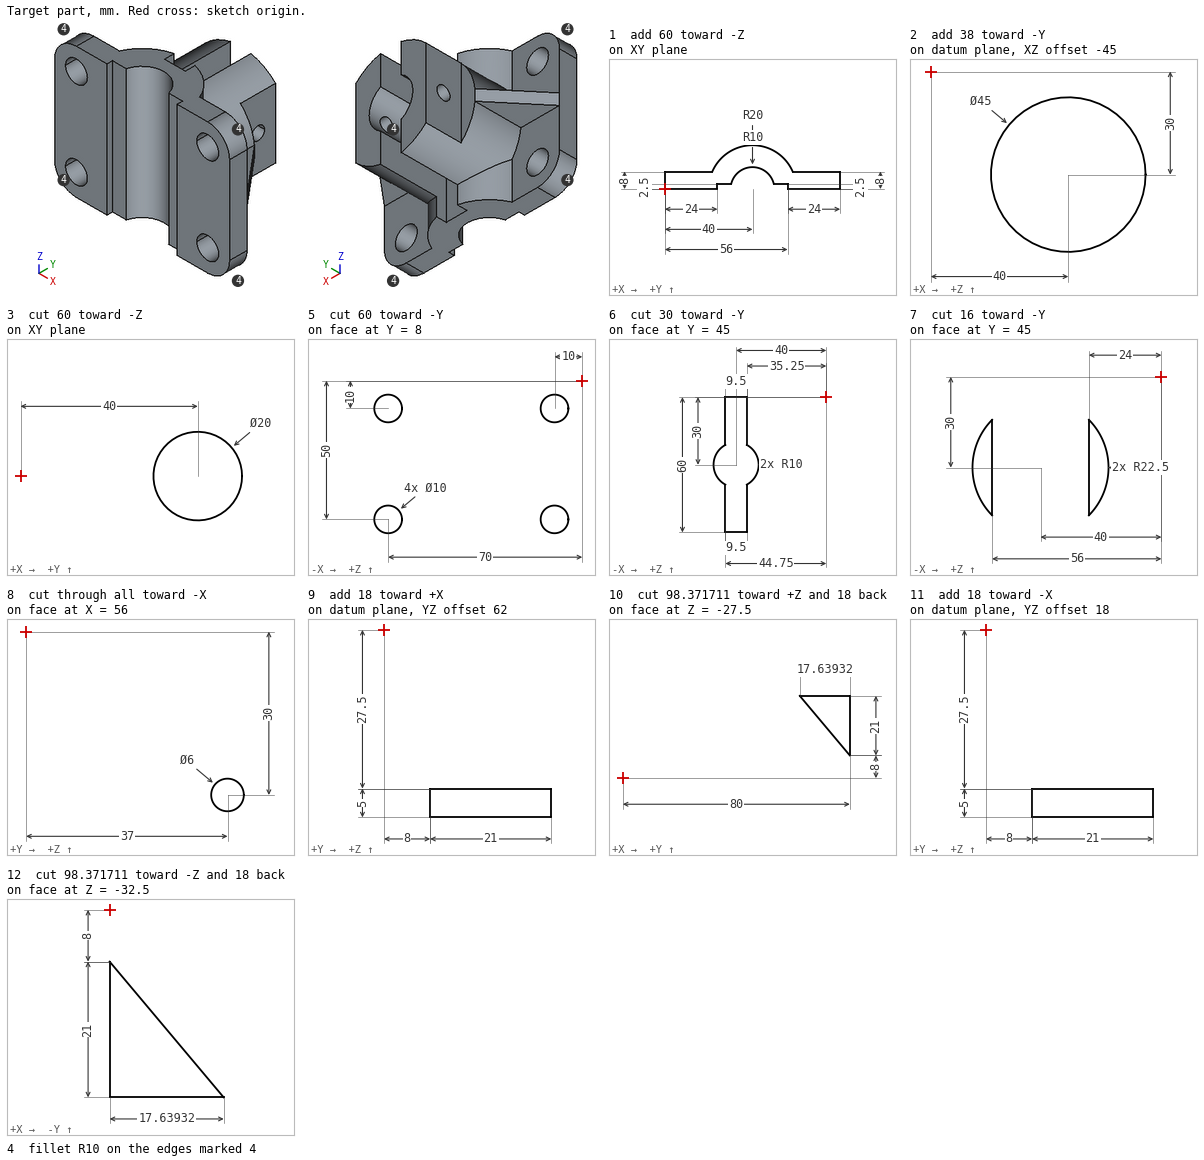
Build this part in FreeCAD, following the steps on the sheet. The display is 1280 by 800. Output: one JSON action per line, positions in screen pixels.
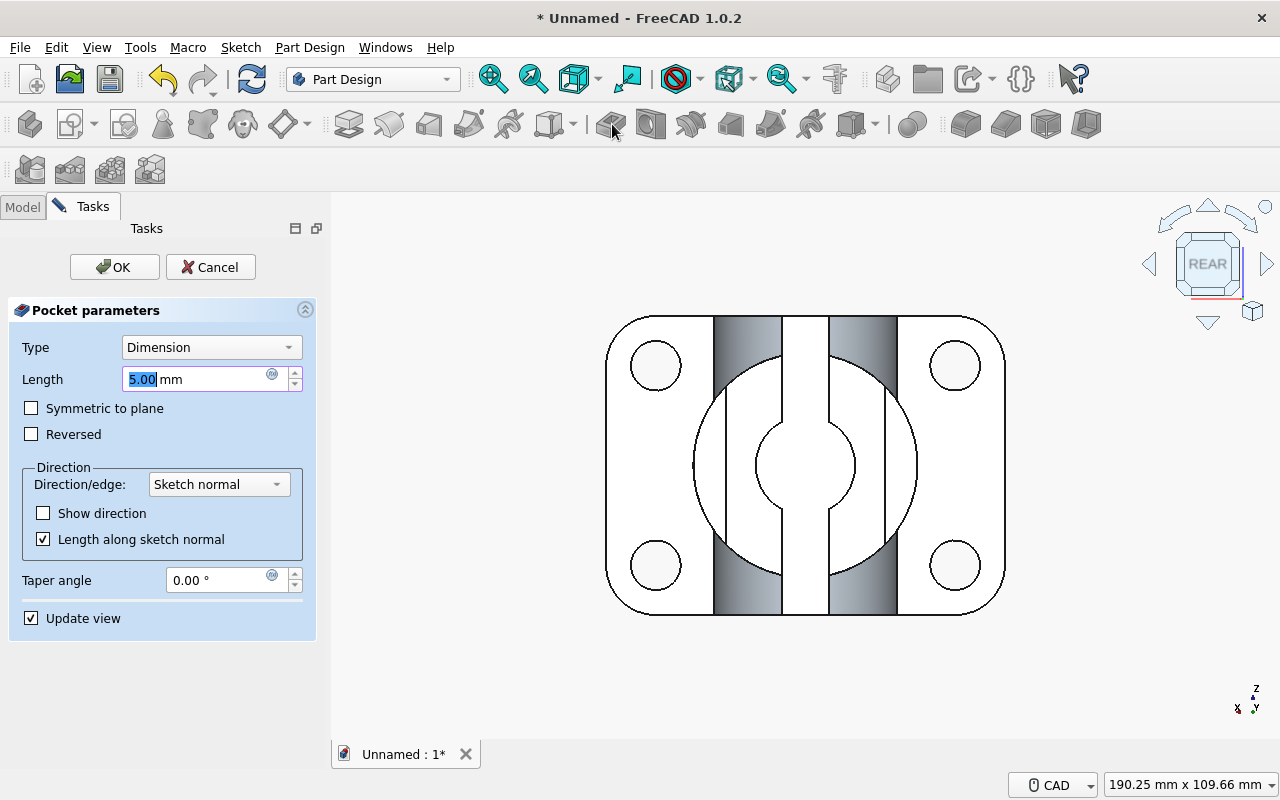
{"action": "type", "text": "16"}
{"action": "key", "text": "Tab"}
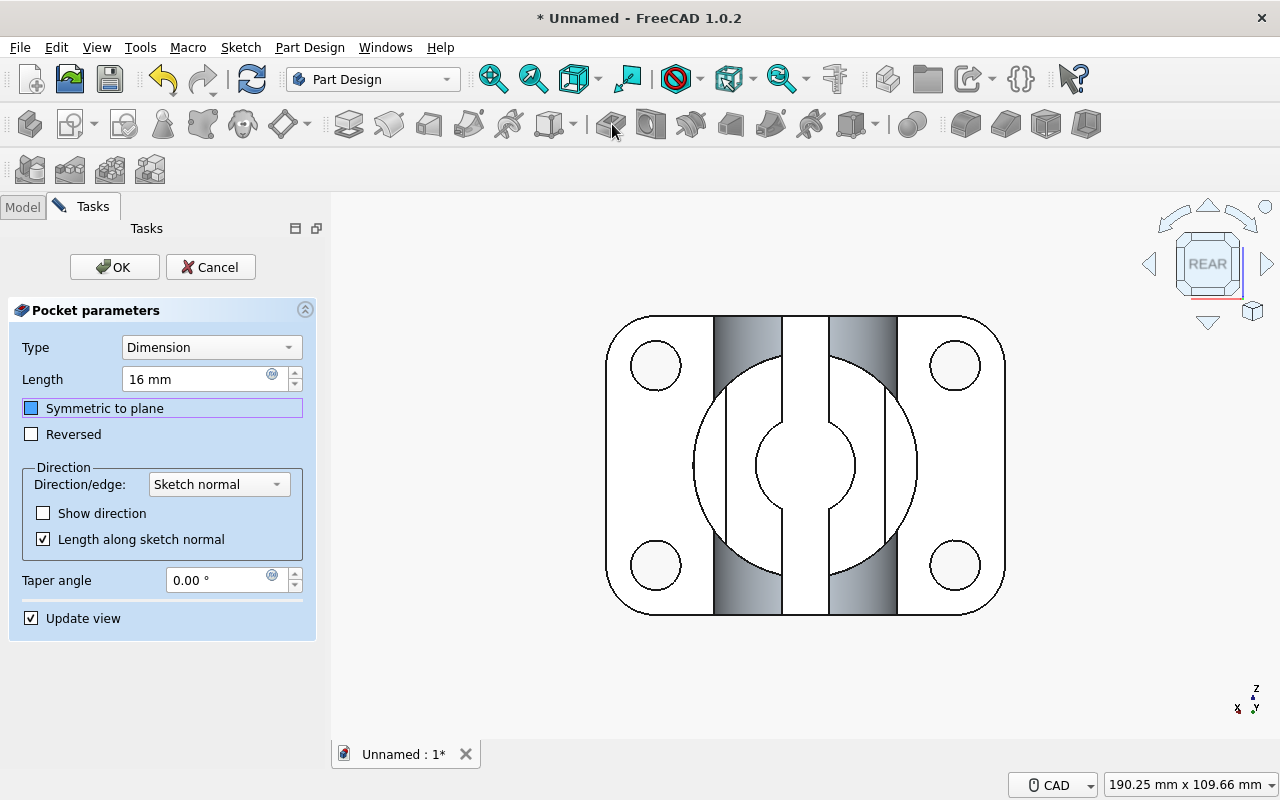
{"action": "left_click", "coordinate": [115, 267]}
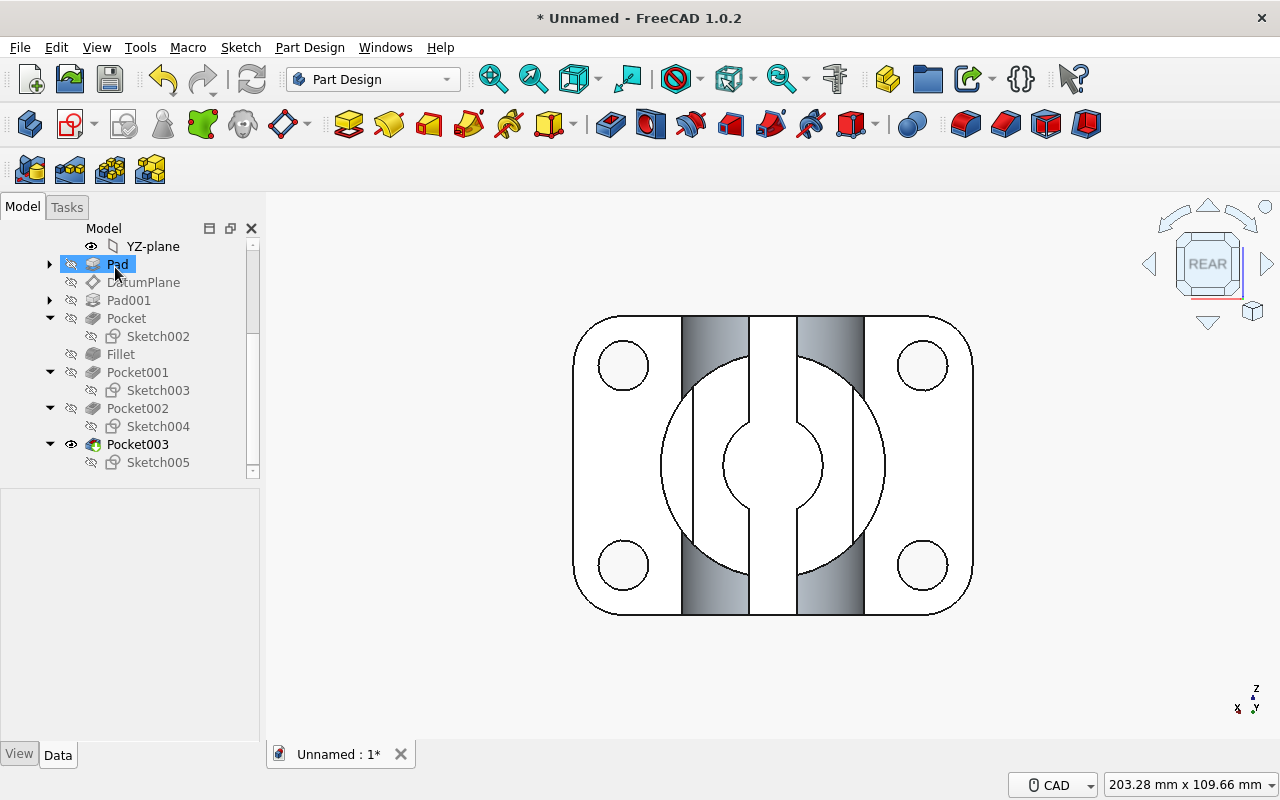
{"action": "key", "text": "0"}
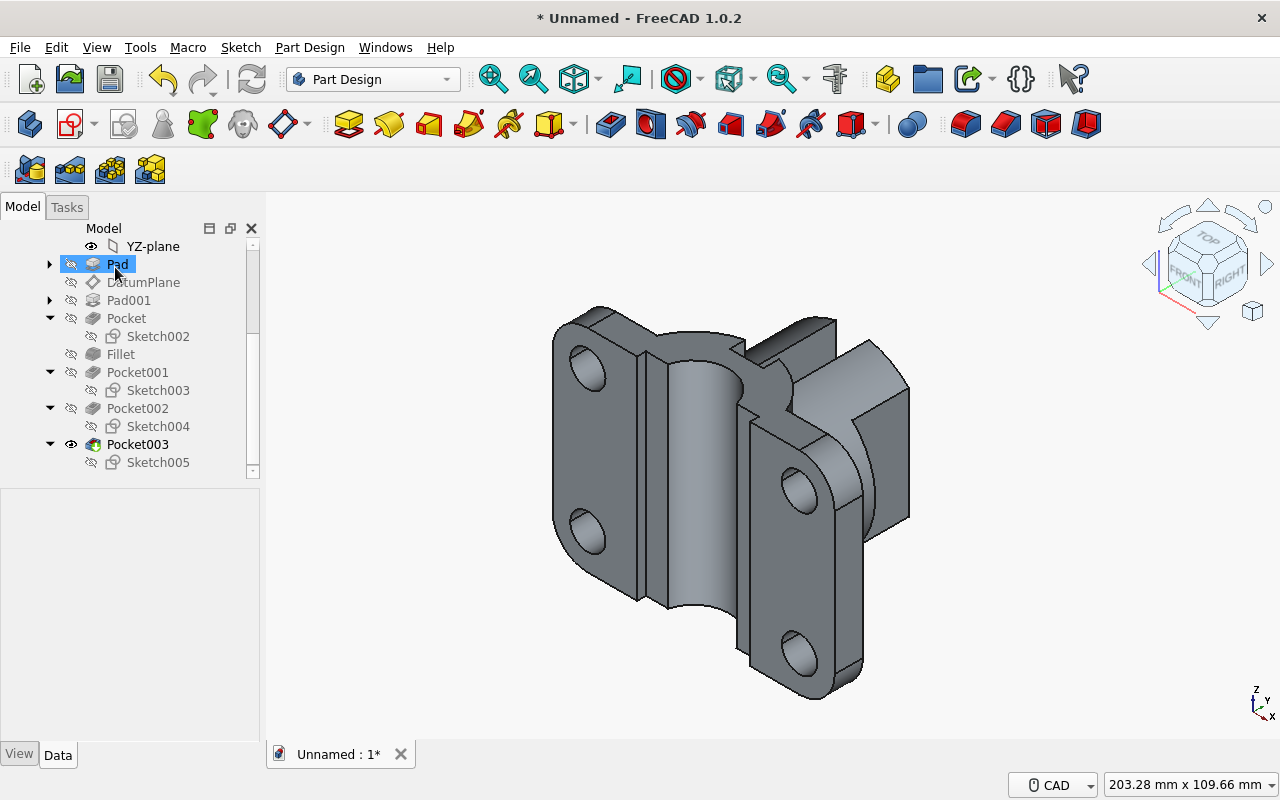
{"action": "left_click", "coordinate": [881, 449]}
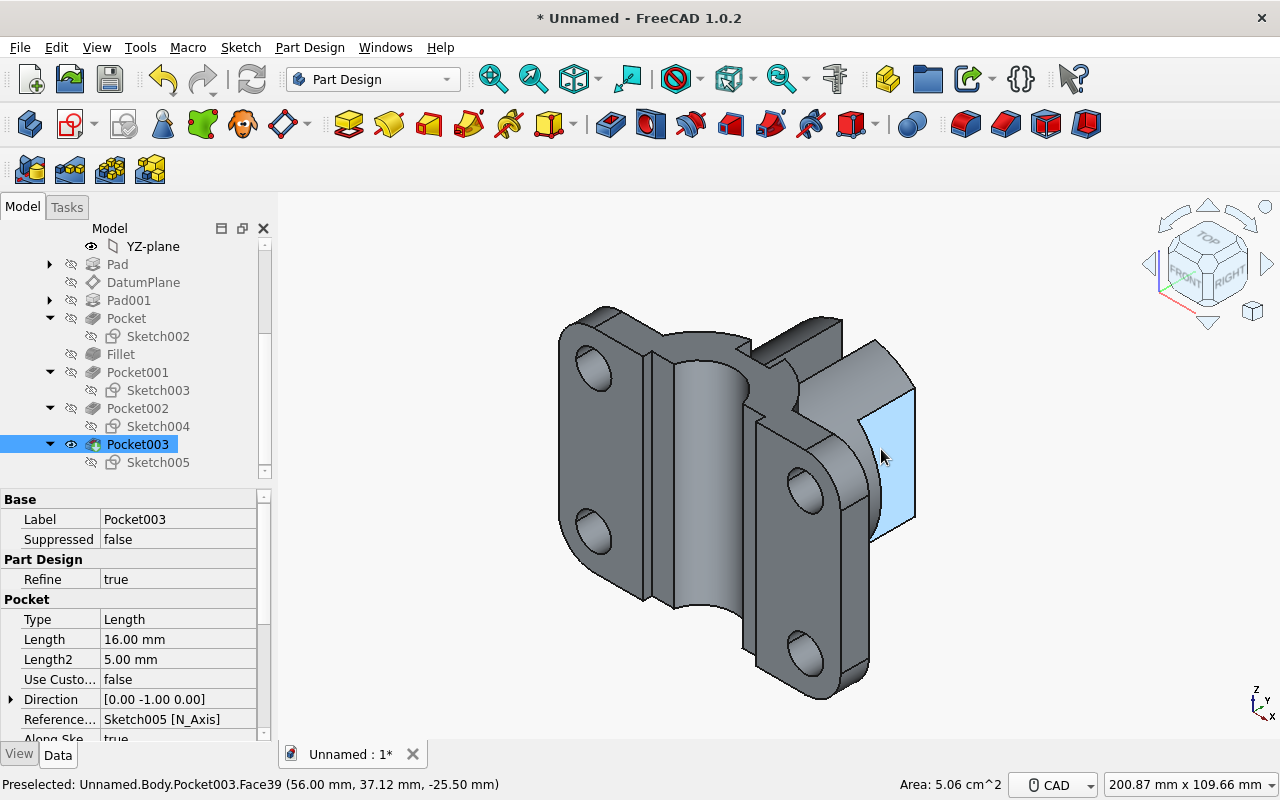
{"action": "left_click", "coordinate": [70, 124]}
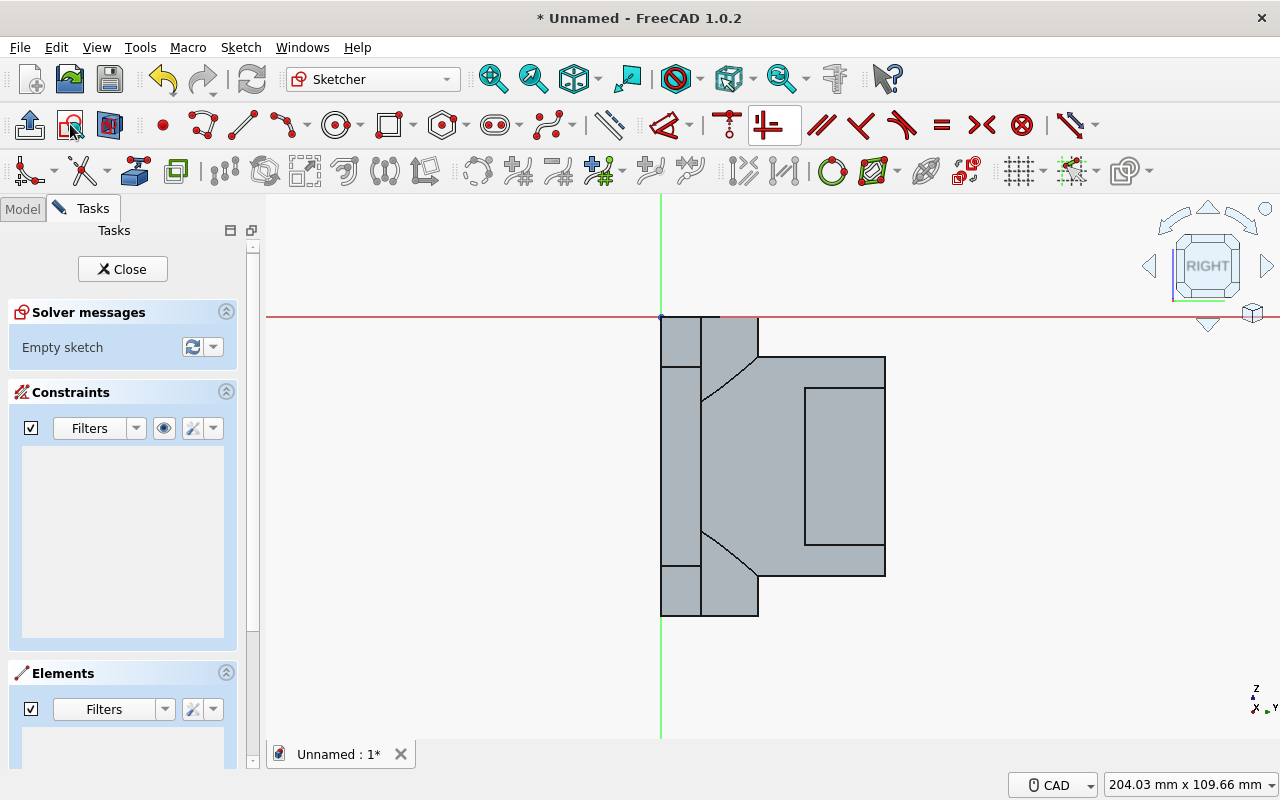
{"action": "scroll", "coordinate": [859, 467], "scroll_direction": "up", "scroll_amount": 12}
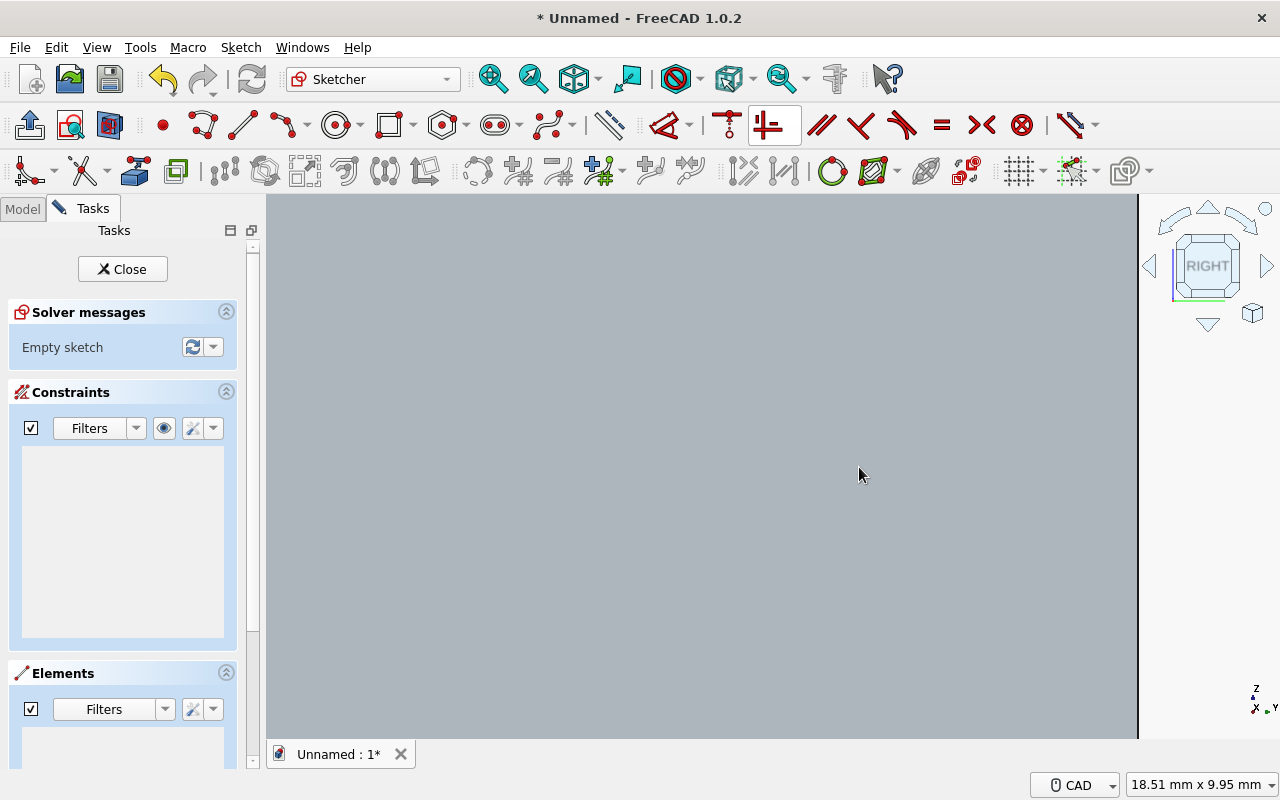
{"action": "left_click", "coordinate": [336, 126]}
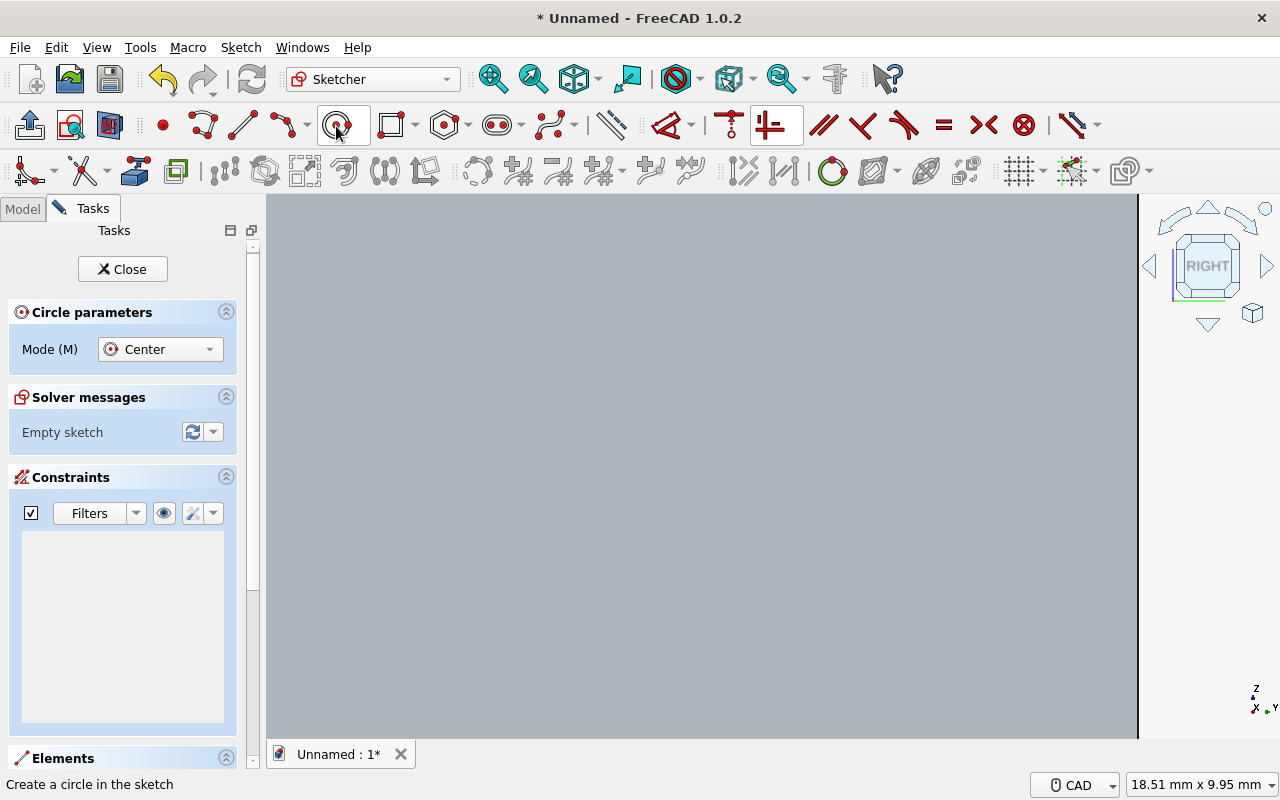
{"action": "left_click", "coordinate": [700, 456]}
{"action": "left_click", "coordinate": [816, 340]}
{"action": "key", "text": "Escape"}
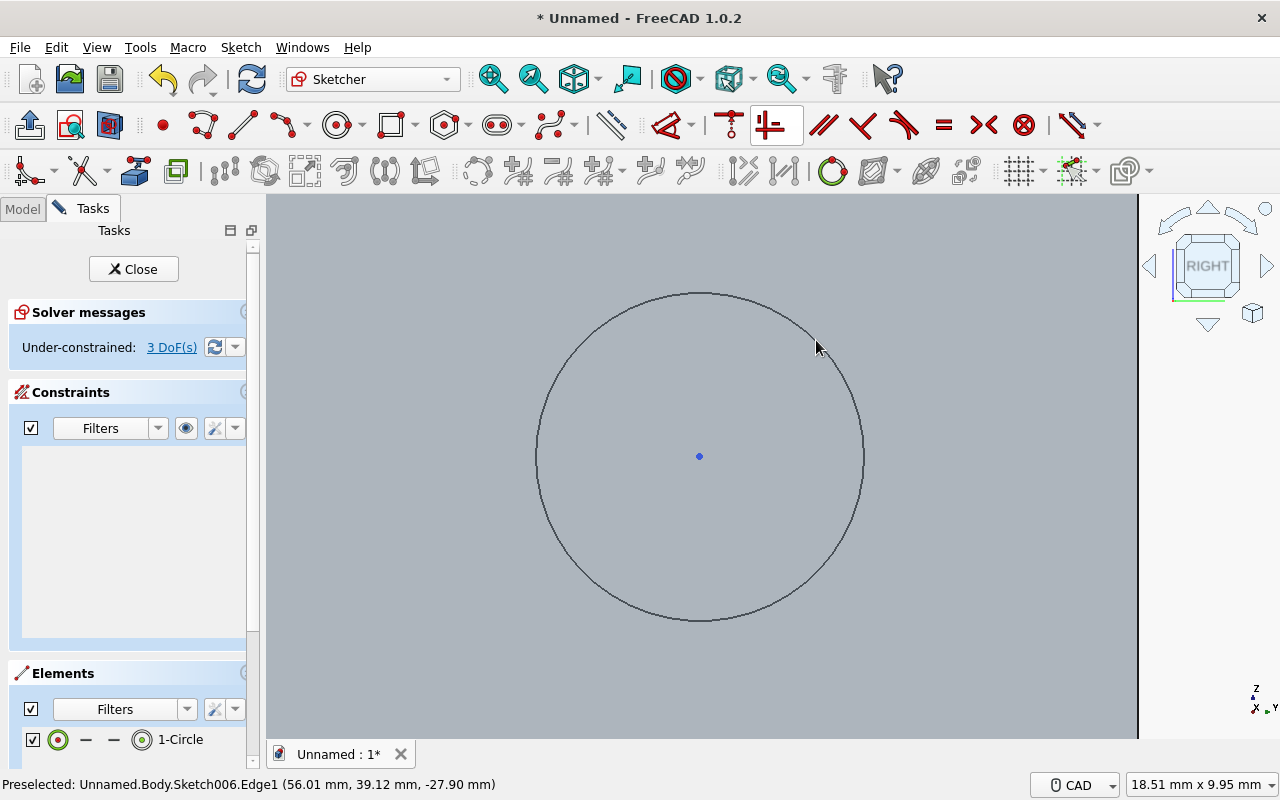
{"action": "left_click", "coordinate": [666, 126]}